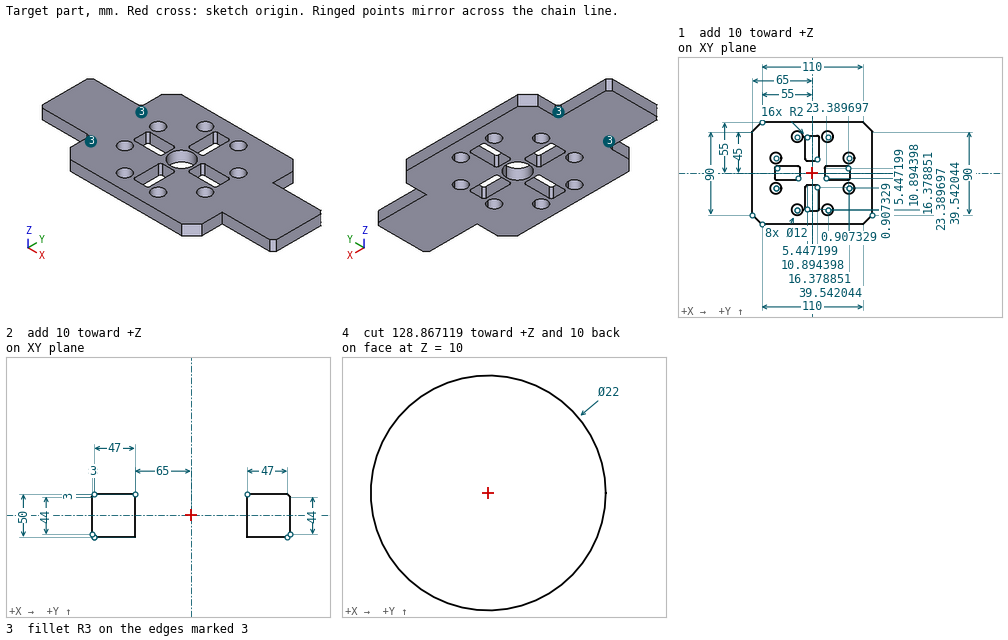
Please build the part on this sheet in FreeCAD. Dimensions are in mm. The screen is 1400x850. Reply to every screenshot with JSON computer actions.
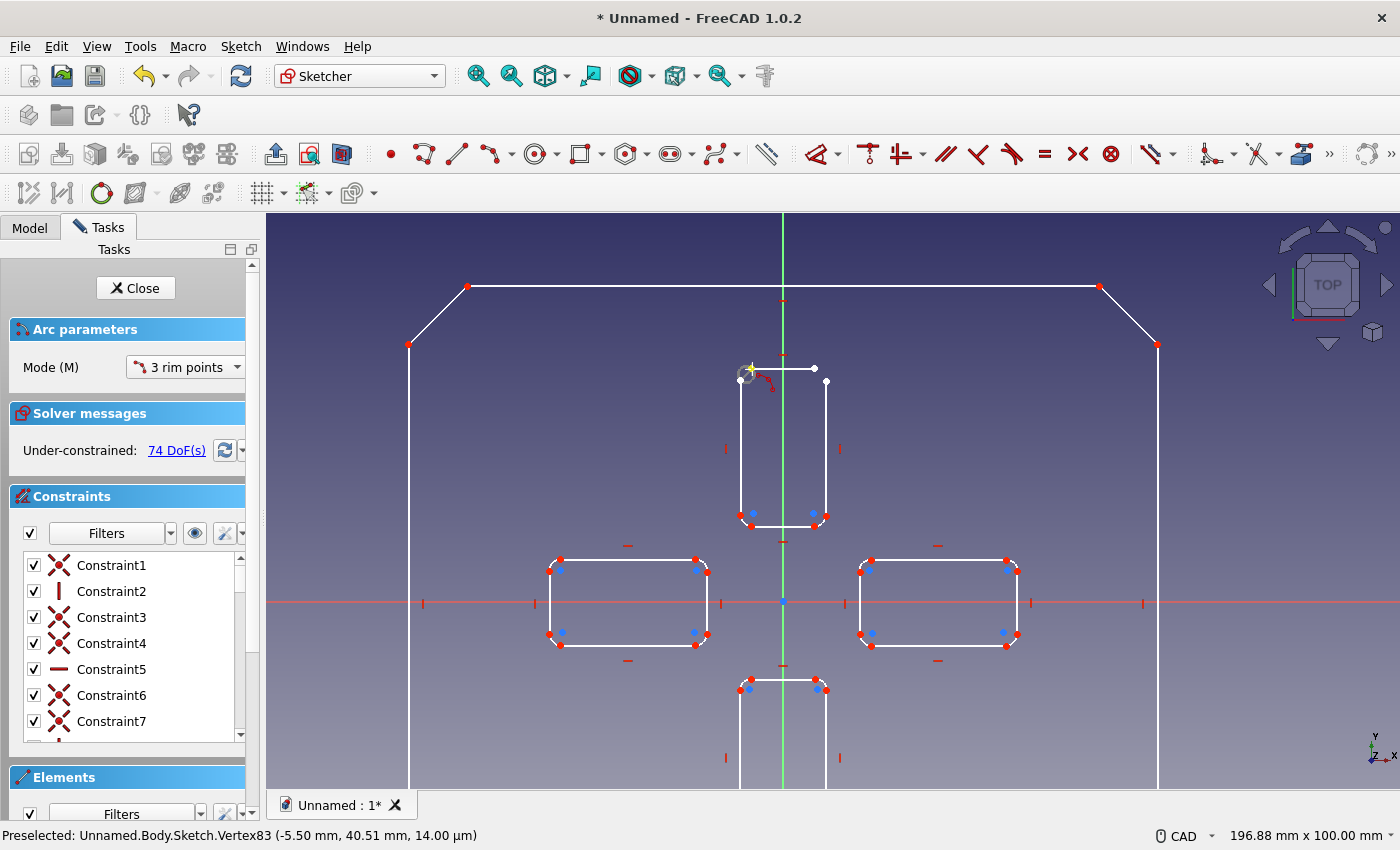
{"action": "scroll", "coordinate": [744, 371], "scroll_direction": "up", "scroll_amount": 8}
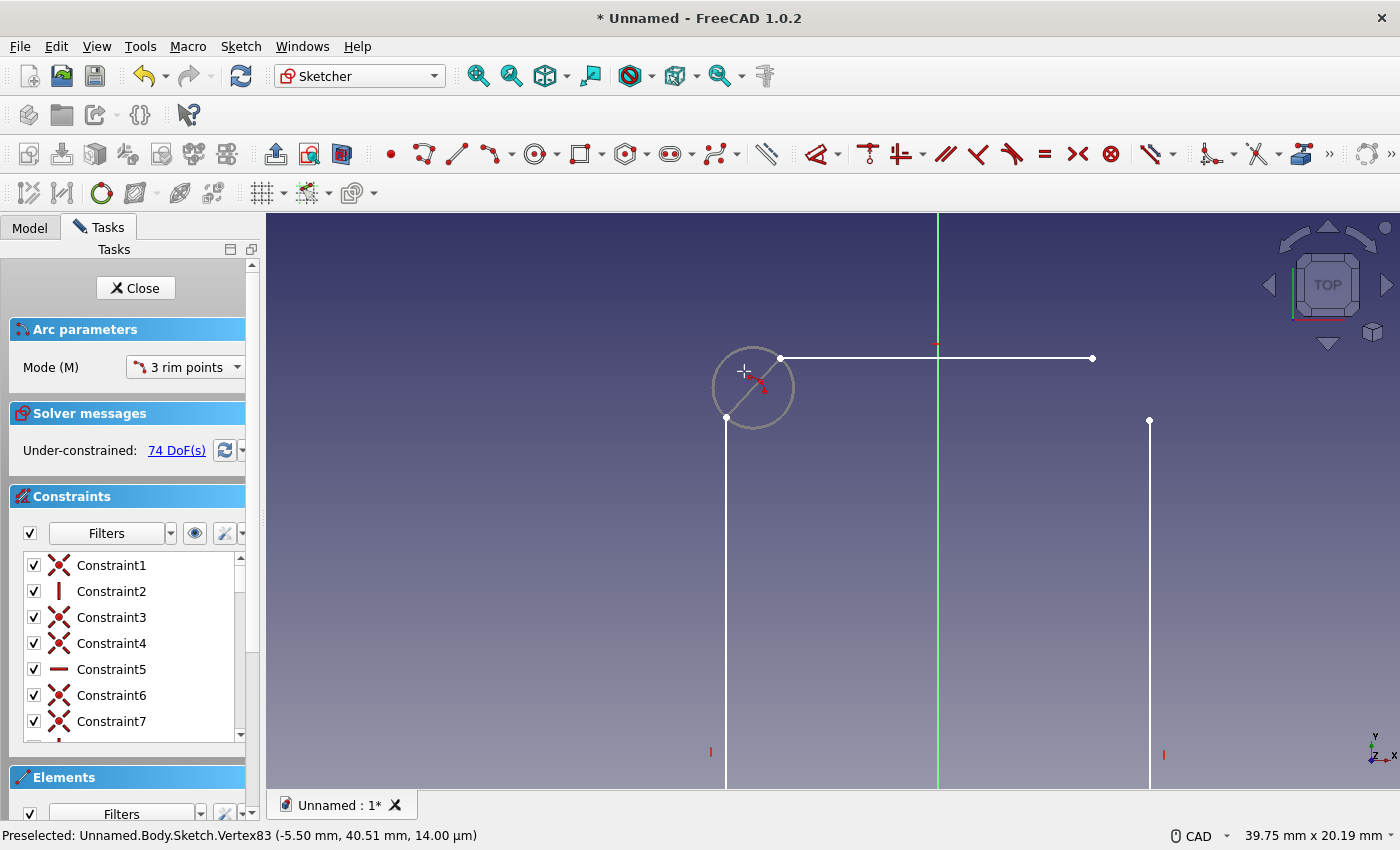
{"action": "left_click", "coordinate": [742, 371]}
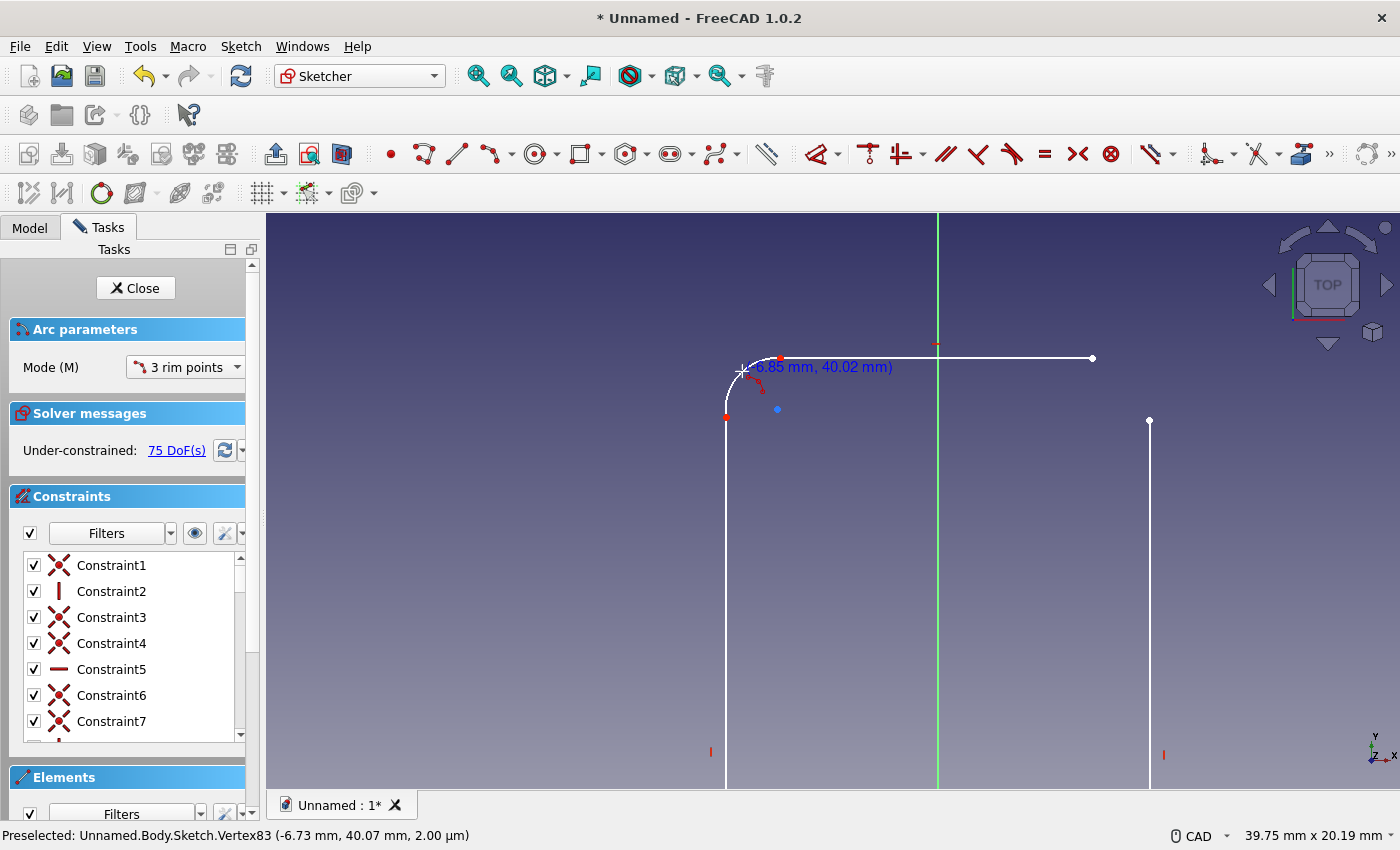
{"action": "scroll", "coordinate": [743, 375], "scroll_direction": "down", "scroll_amount": 11}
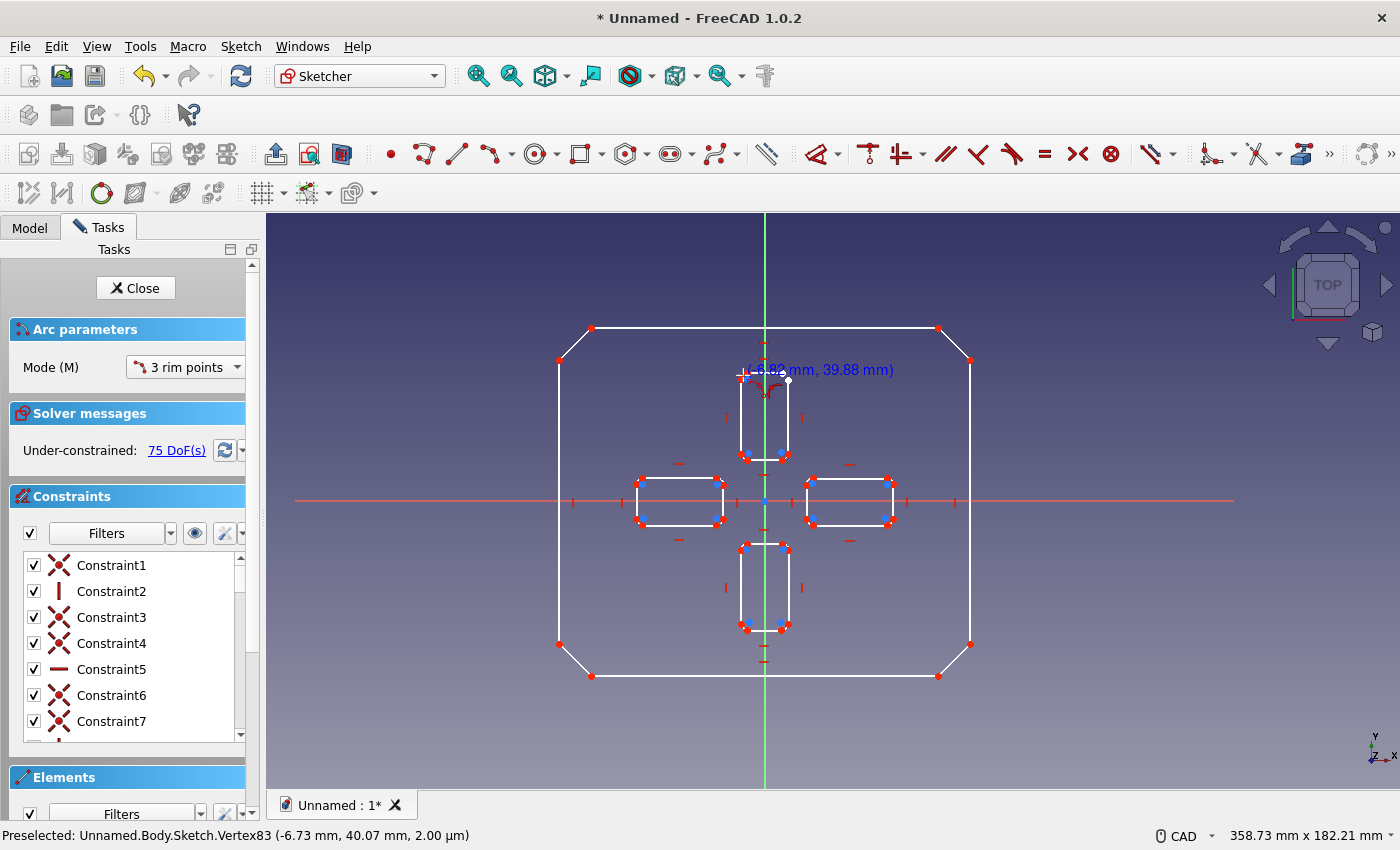
{"action": "scroll", "coordinate": [782, 373], "scroll_direction": "up", "scroll_amount": 3}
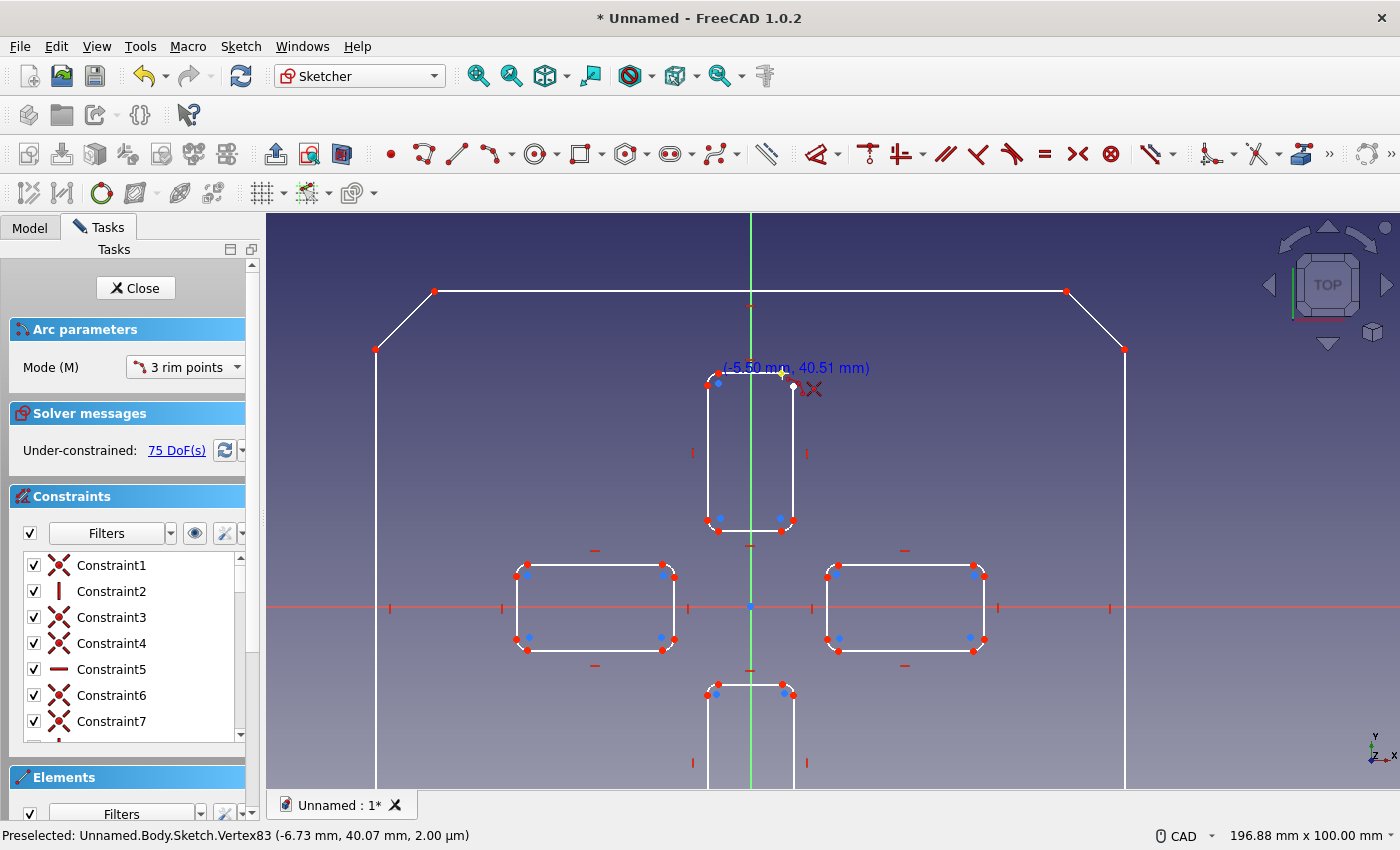
{"action": "left_click", "coordinate": [782, 373]}
{"action": "left_click", "coordinate": [793, 386]}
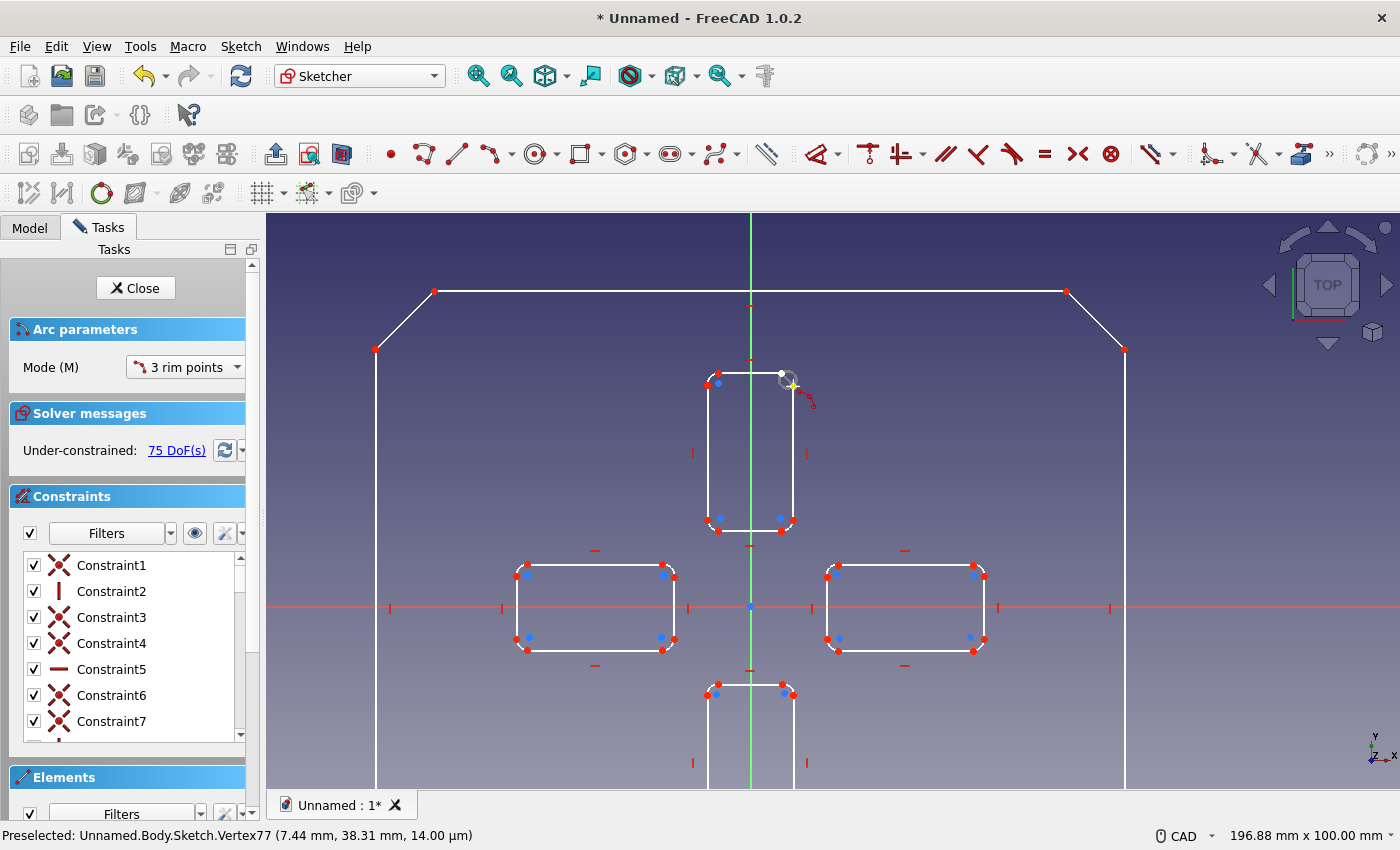
{"action": "scroll", "coordinate": [790, 376], "scroll_direction": "up", "scroll_amount": 8}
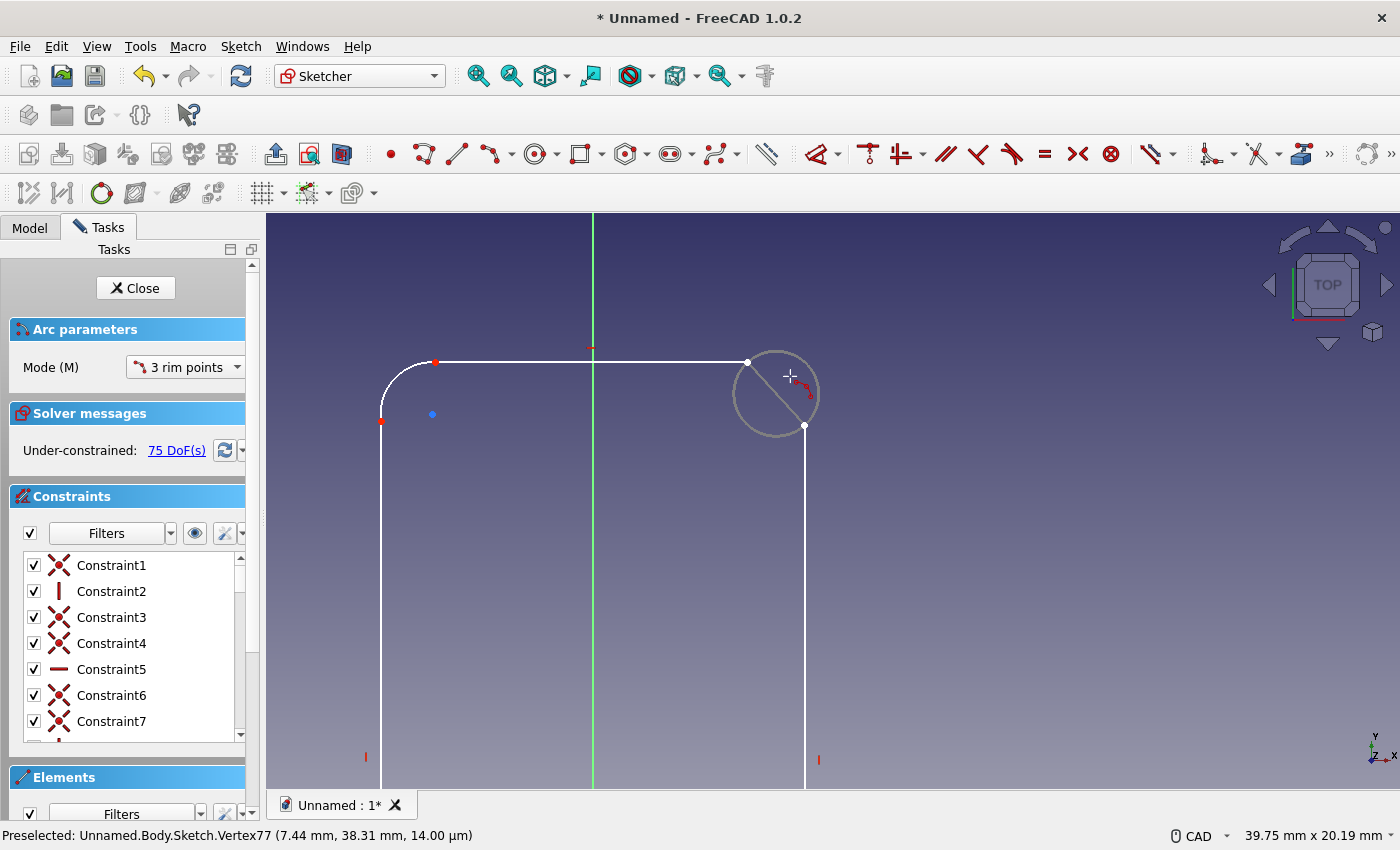
{"action": "left_click", "coordinate": [788, 375]}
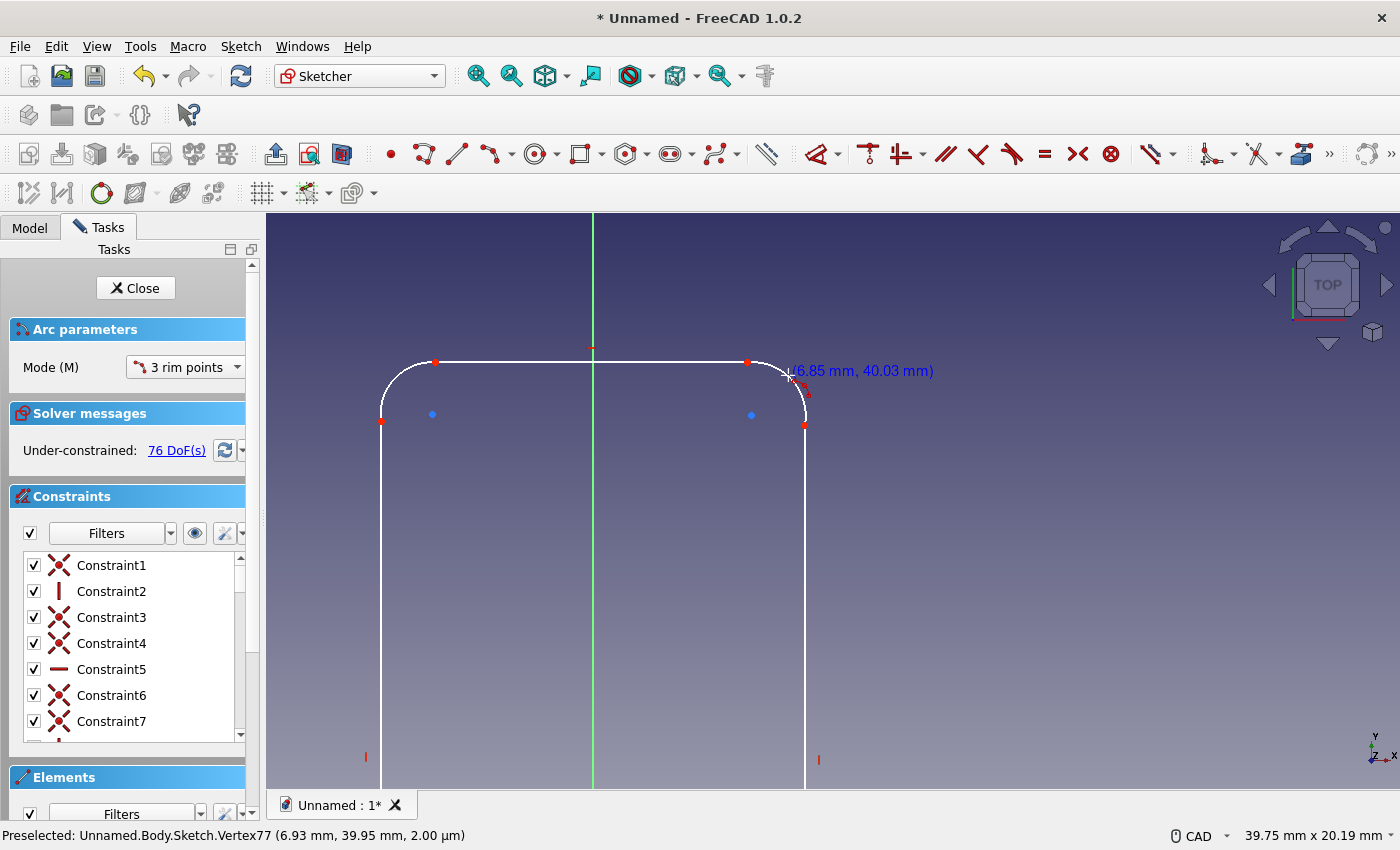
{"action": "left_click", "coordinate": [534, 154]}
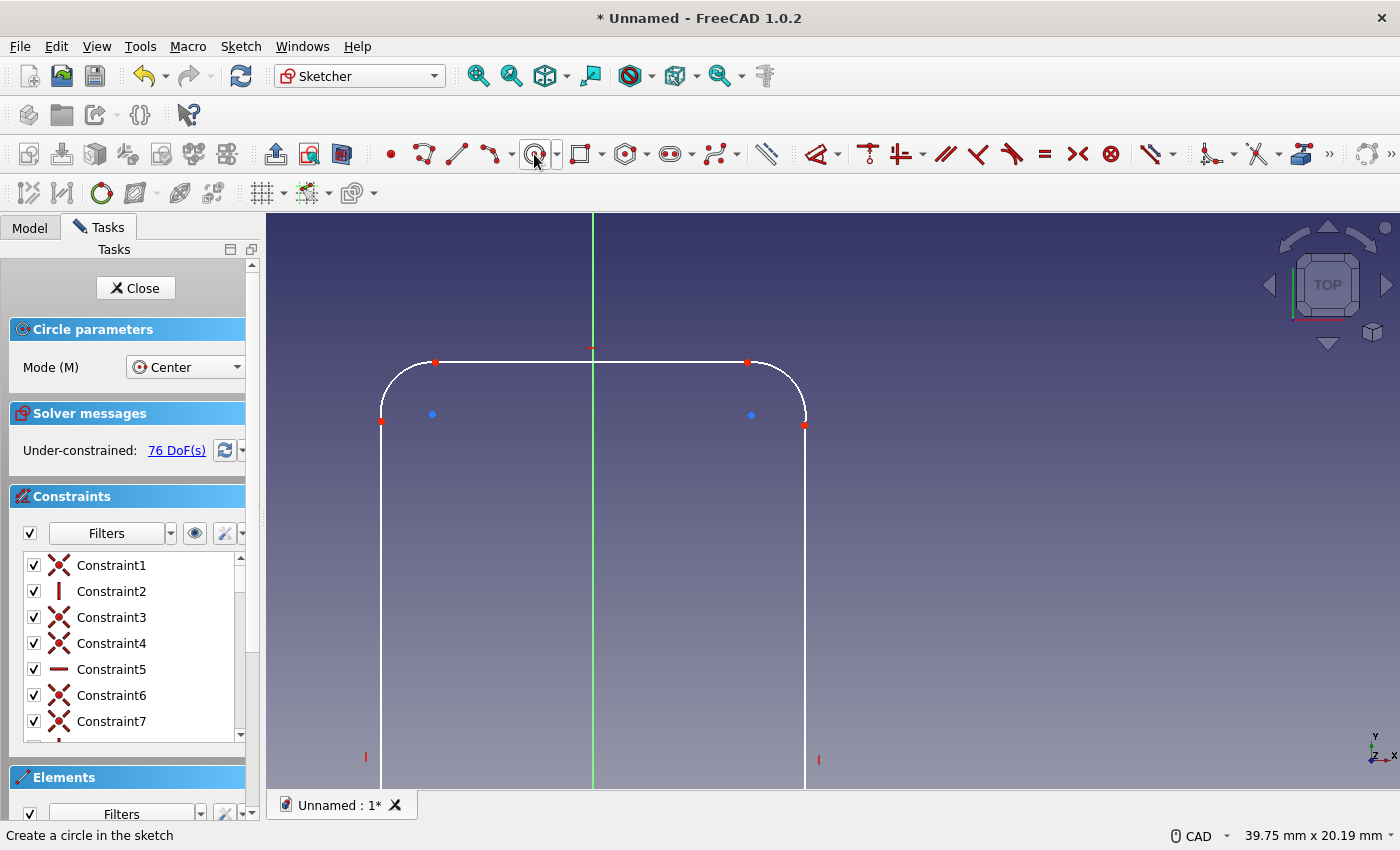
{"action": "scroll", "coordinate": [786, 374], "scroll_direction": "down", "scroll_amount": 11}